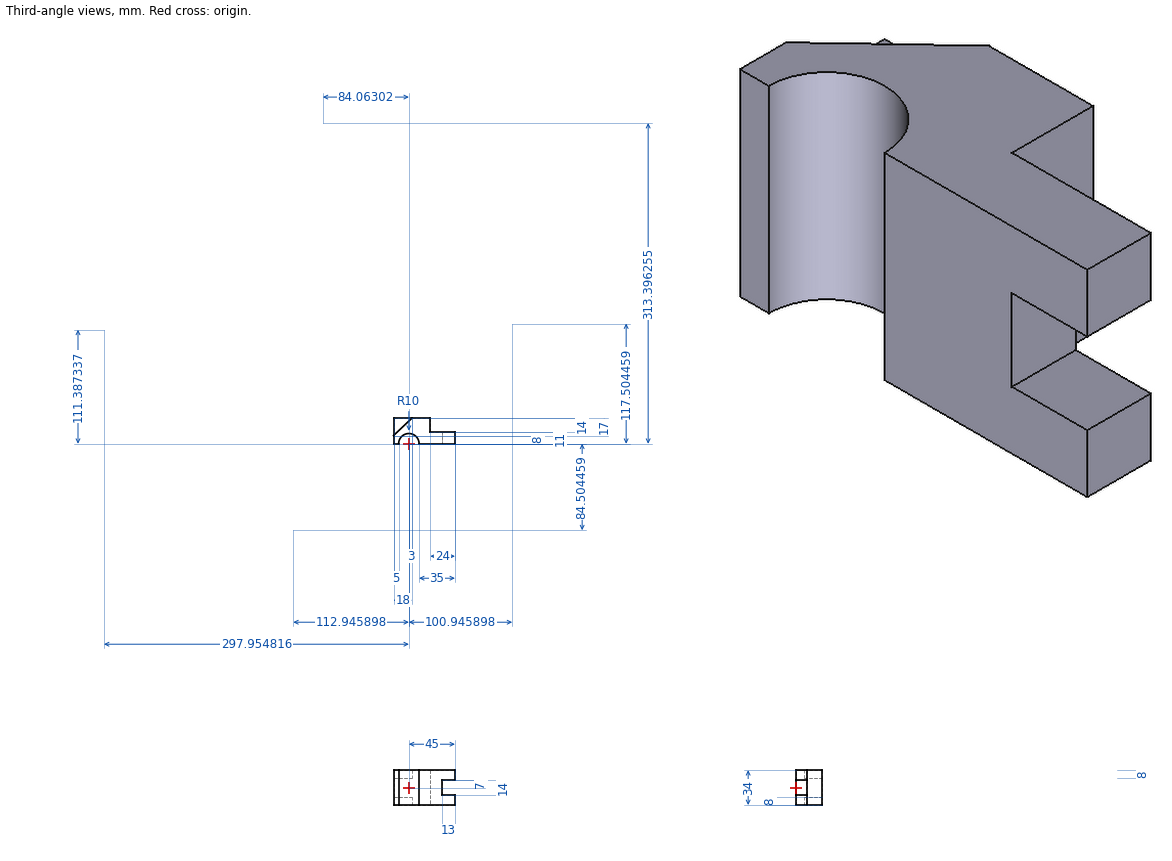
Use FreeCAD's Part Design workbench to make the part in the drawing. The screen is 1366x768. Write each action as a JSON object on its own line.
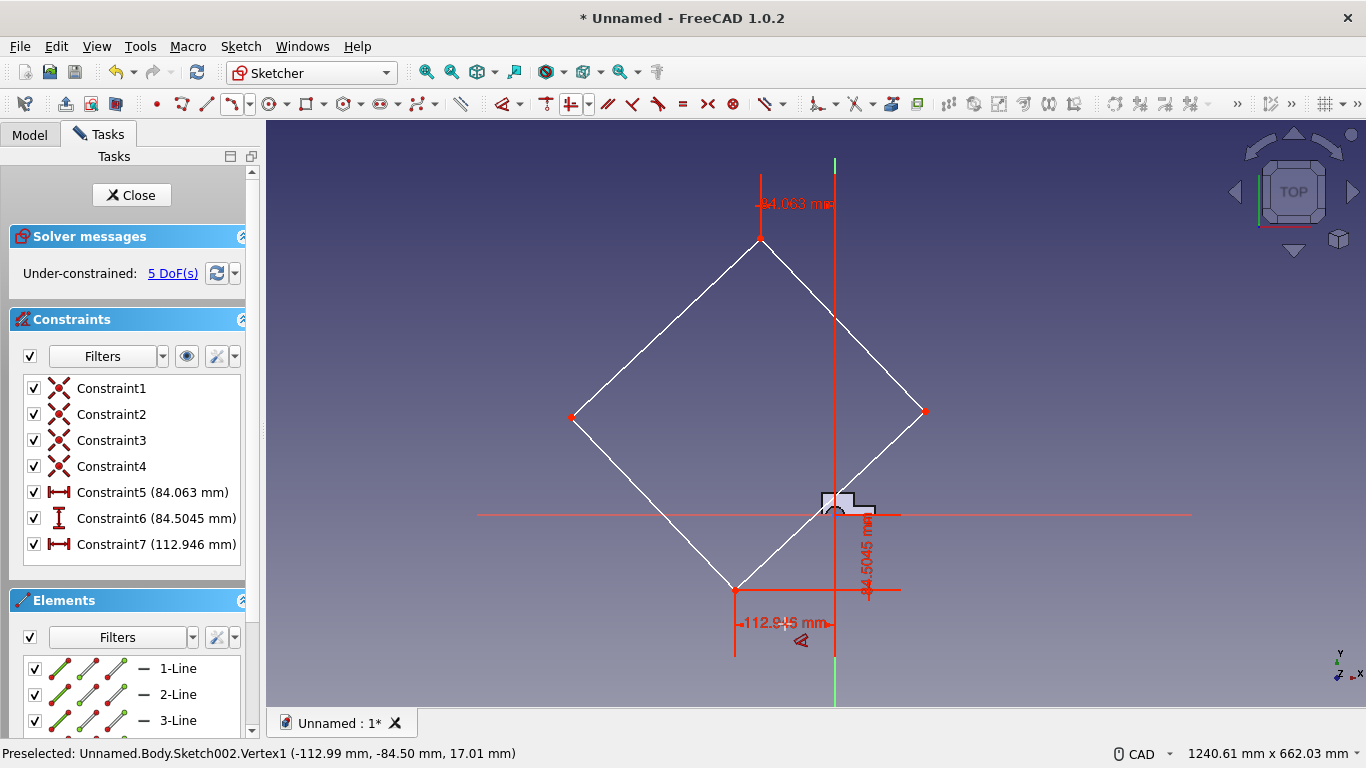
{"action": "left_click", "coordinate": [925, 412]}
{"action": "left_click", "coordinate": [859, 378]}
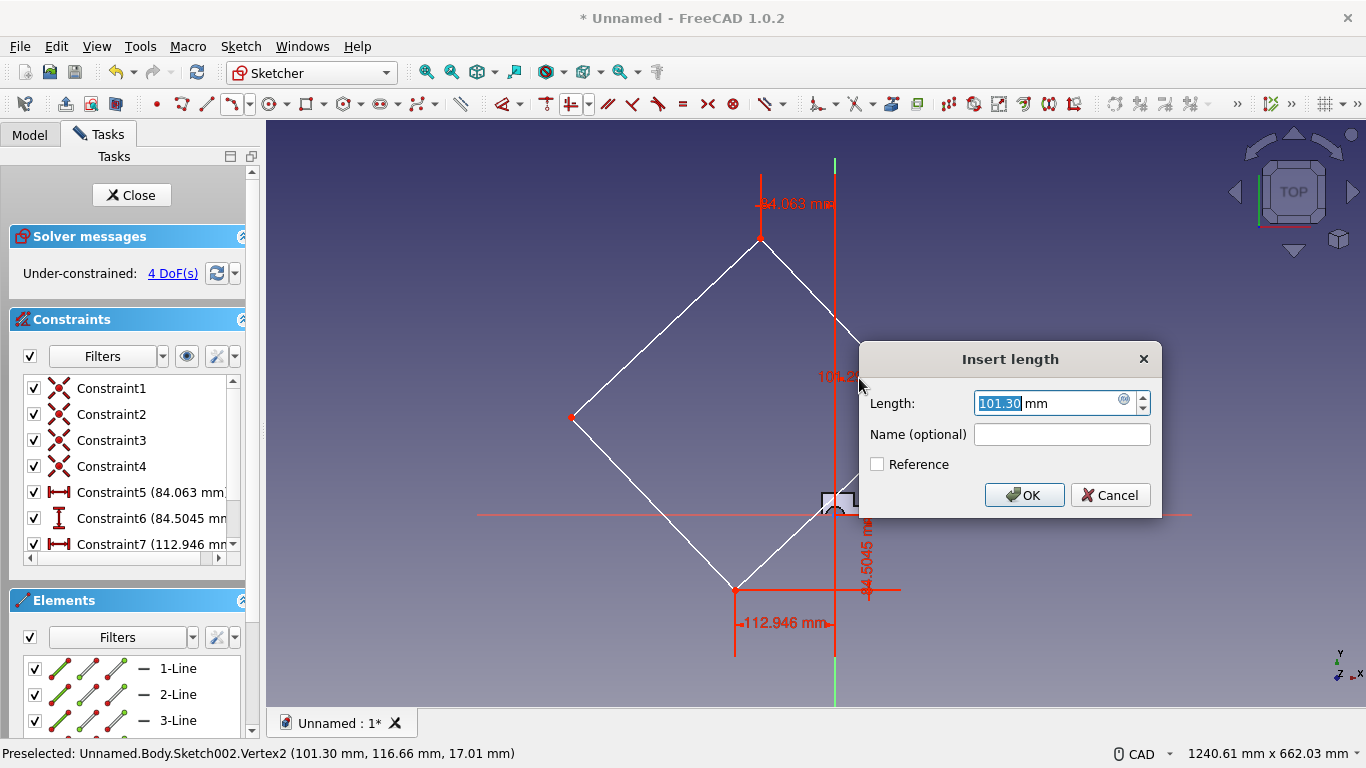
{"action": "type", "text": "100.945898"}
{"action": "key", "text": "Return"}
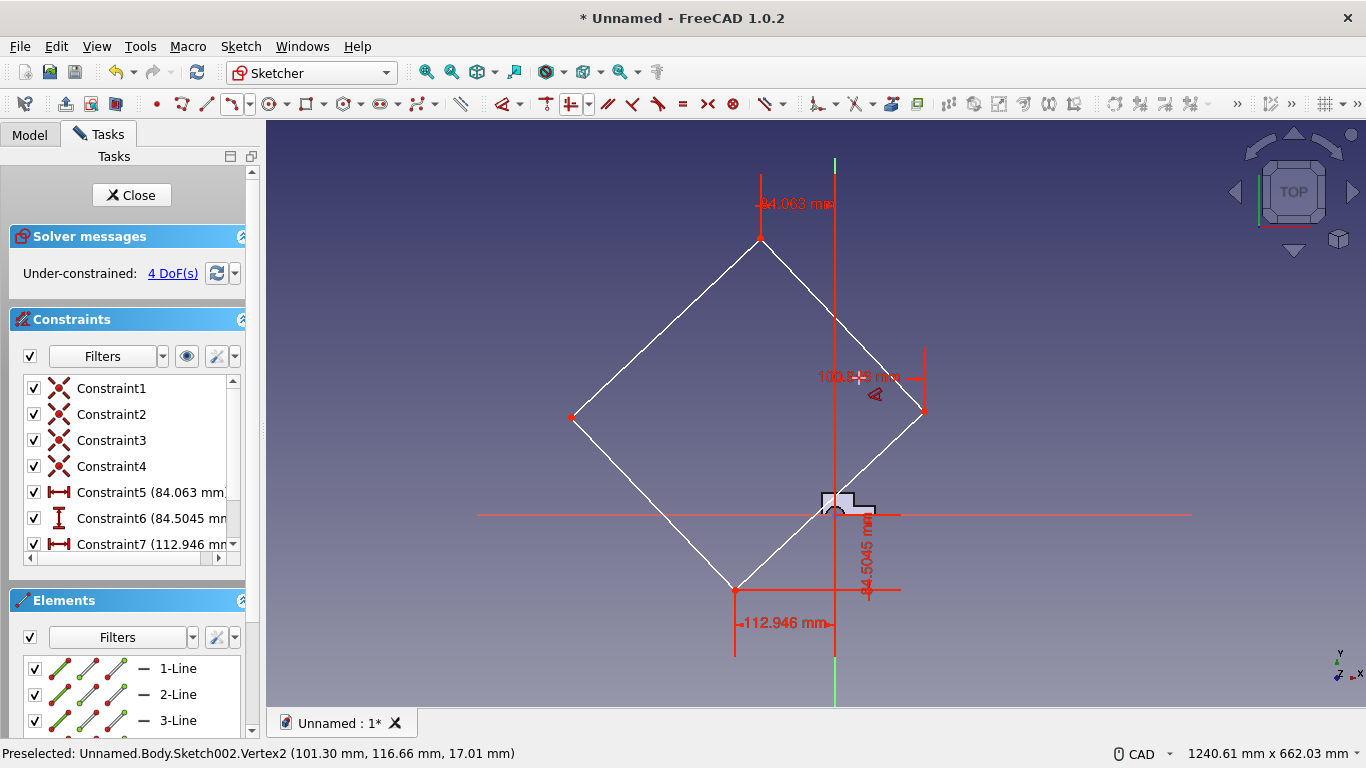
{"action": "left_click", "coordinate": [925, 412]}
{"action": "left_click", "coordinate": [959, 464]}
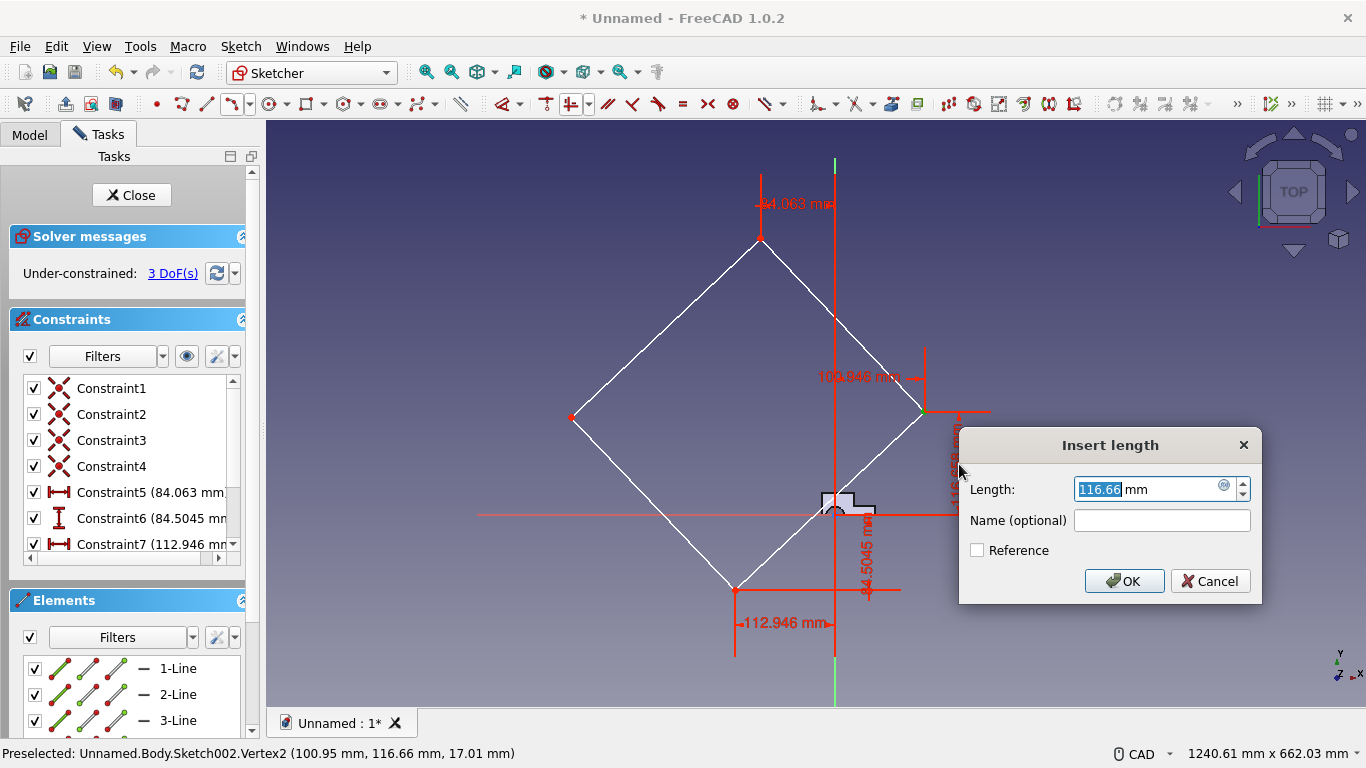
{"action": "type", "text": "117.504459"}
{"action": "key", "text": "Return"}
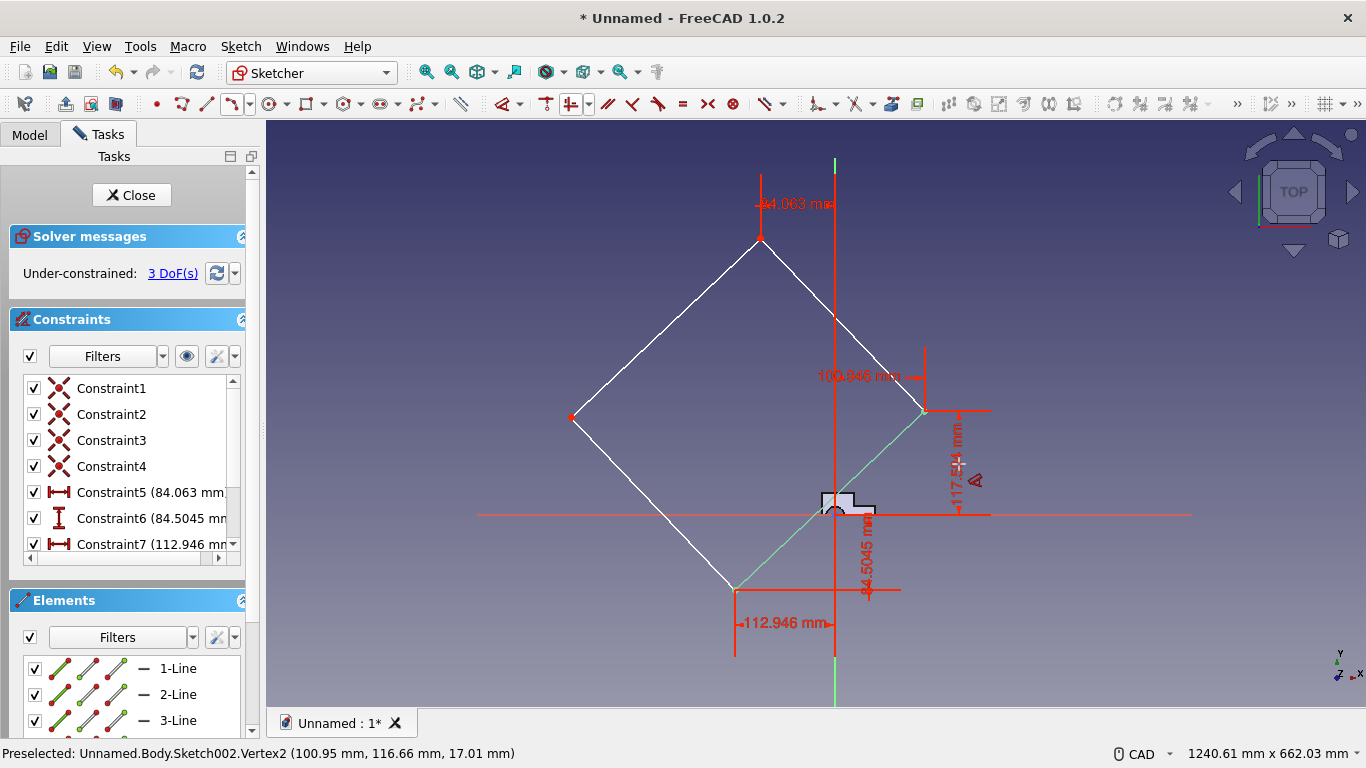
{"action": "left_click", "coordinate": [761, 239]}
{"action": "left_click", "coordinate": [869, 314]}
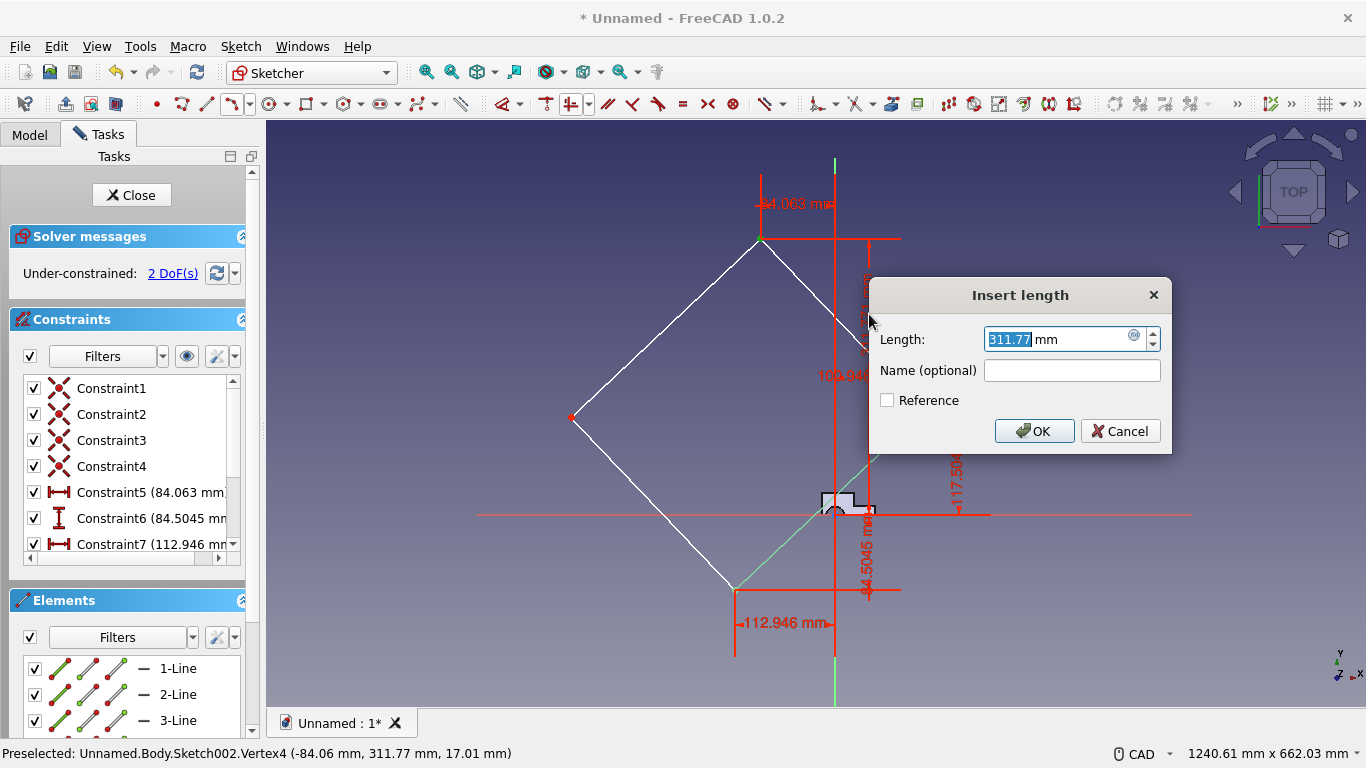
{"action": "type", "text": "313.396255"}
{"action": "key", "text": "Return"}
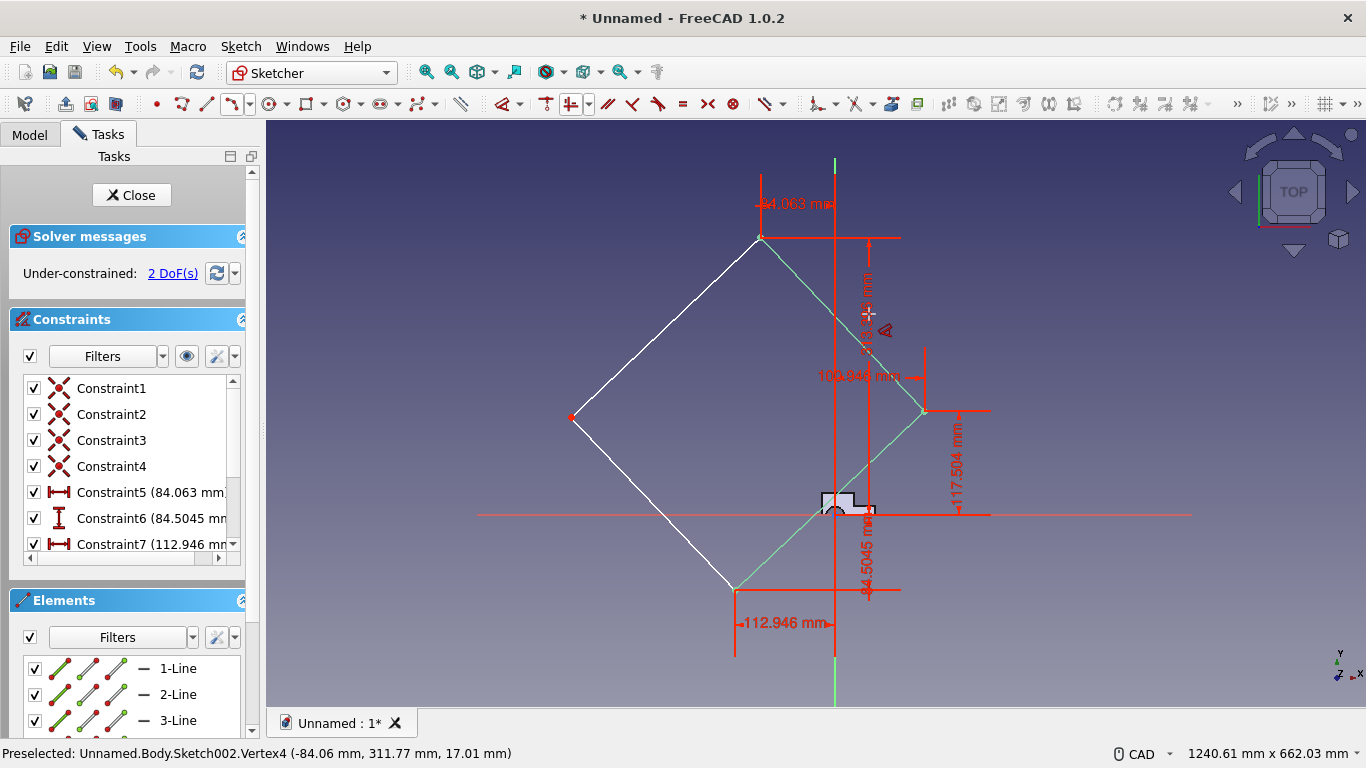
{"action": "left_click", "coordinate": [571, 418]}
{"action": "left_click", "coordinate": [642, 549]}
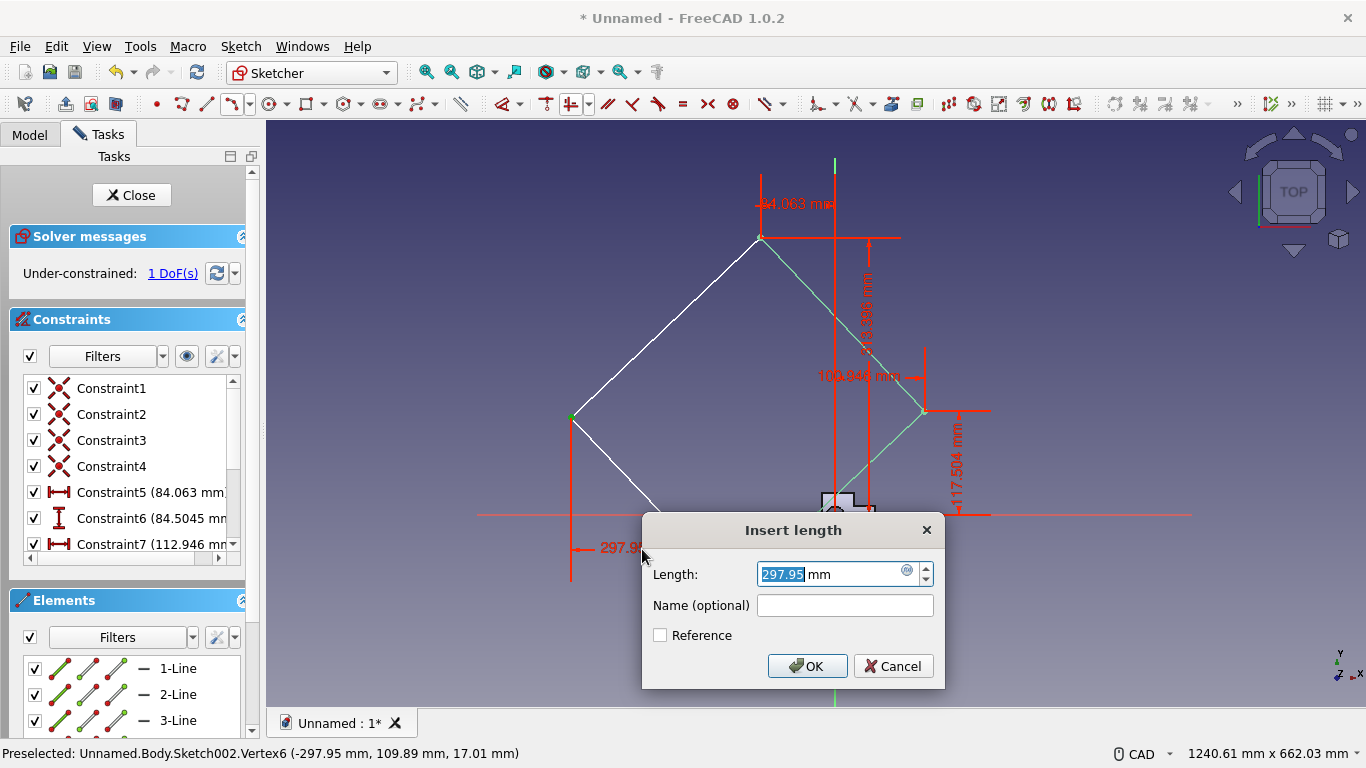
{"action": "type", "text": "297.954816"}
{"action": "key", "text": "Return"}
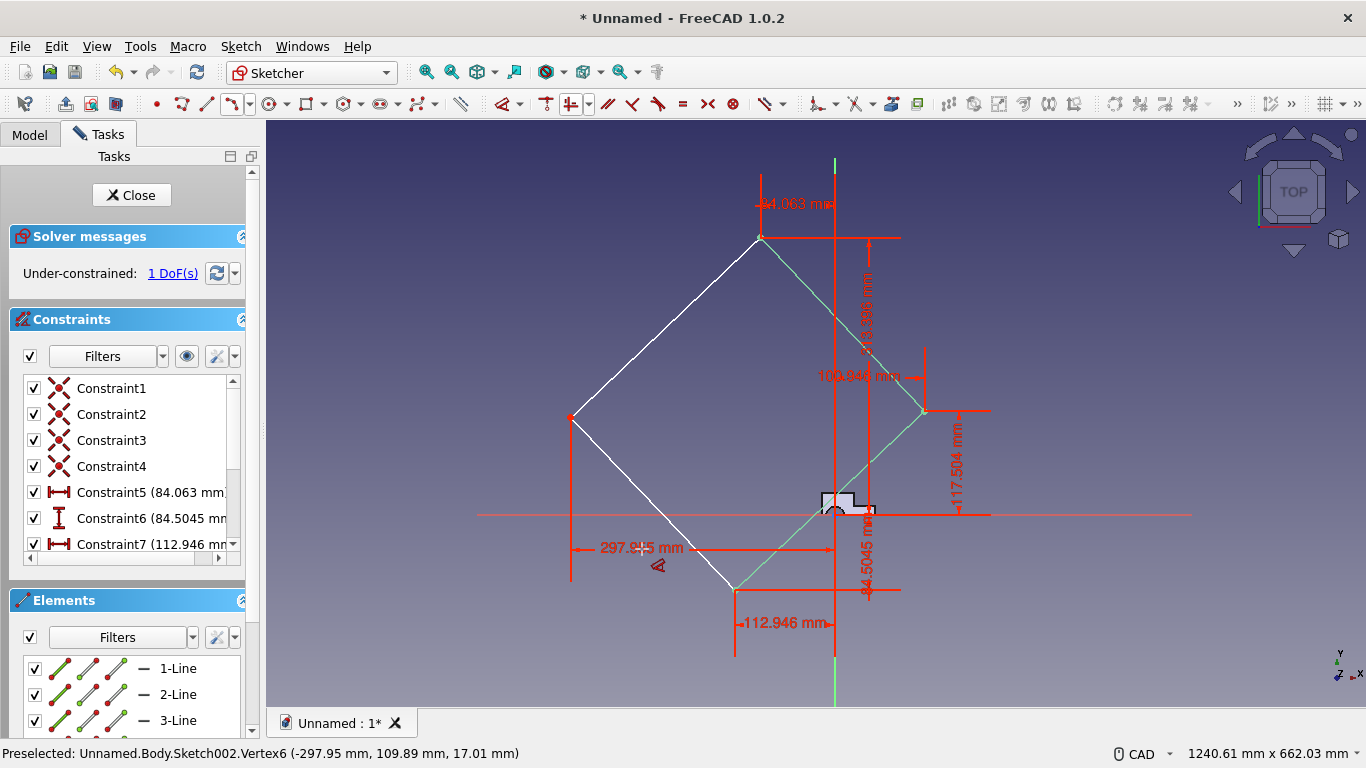
{"action": "left_click", "coordinate": [571, 418]}
{"action": "left_click", "coordinate": [537, 467]}